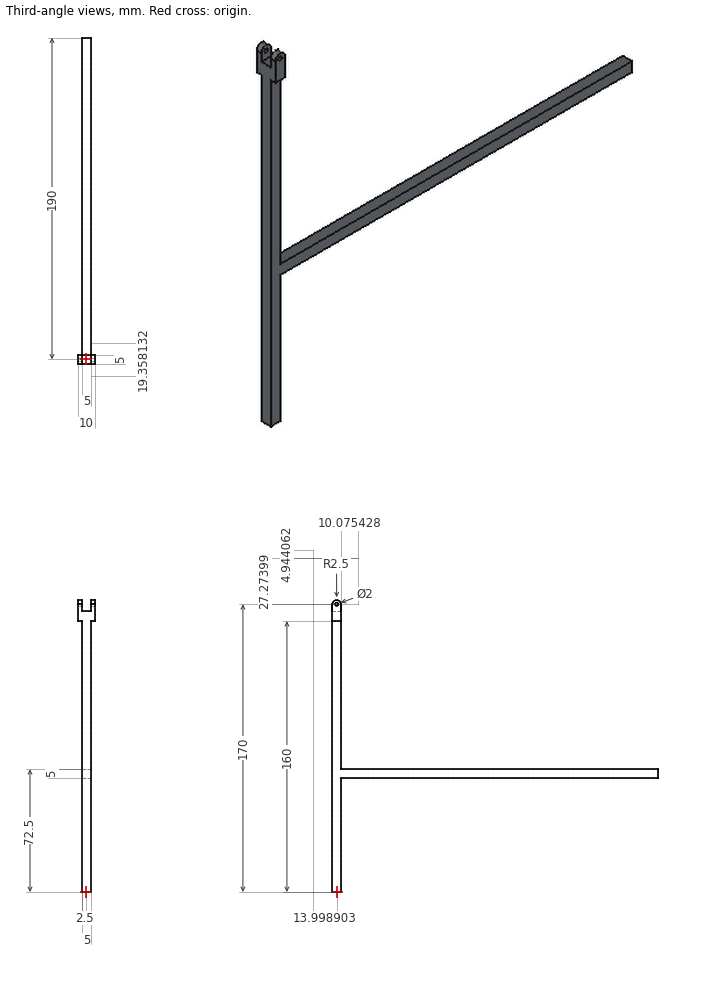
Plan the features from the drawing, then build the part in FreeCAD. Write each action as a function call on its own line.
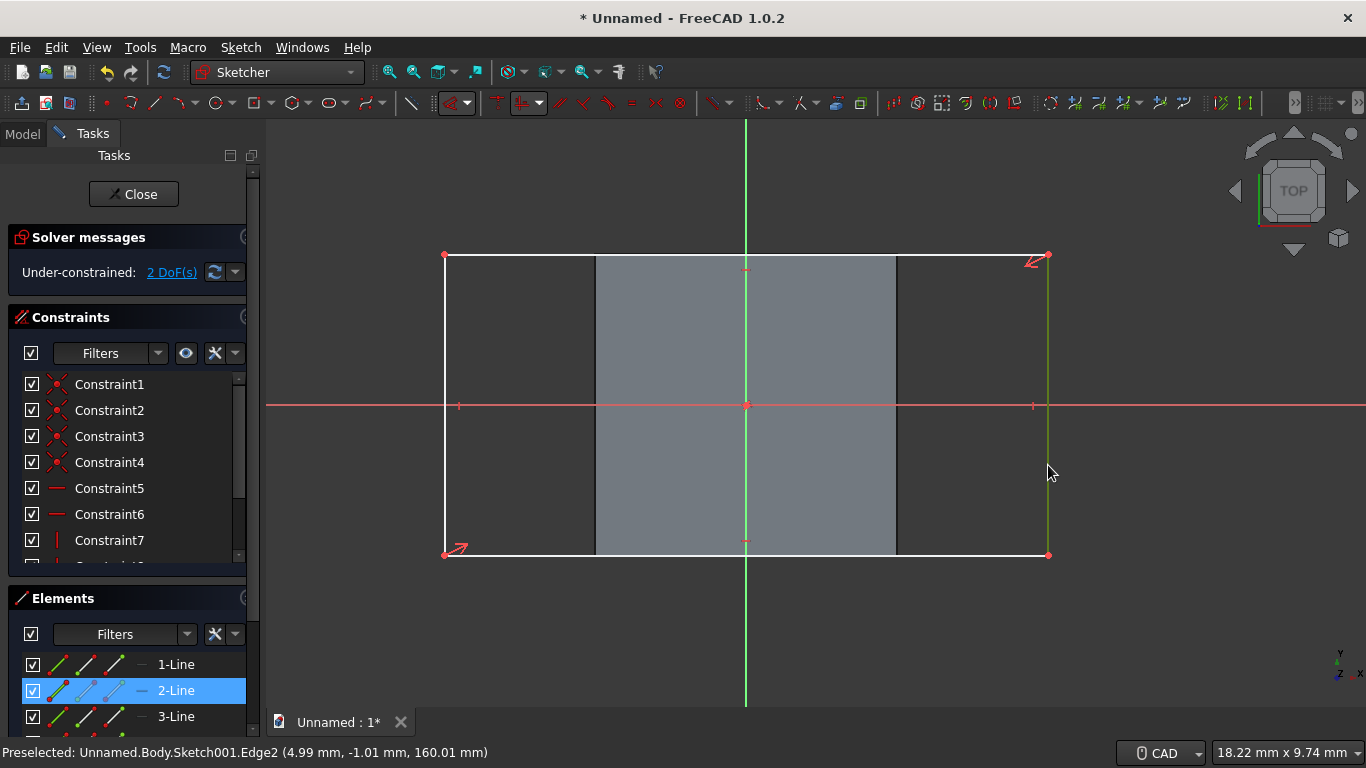
key(i)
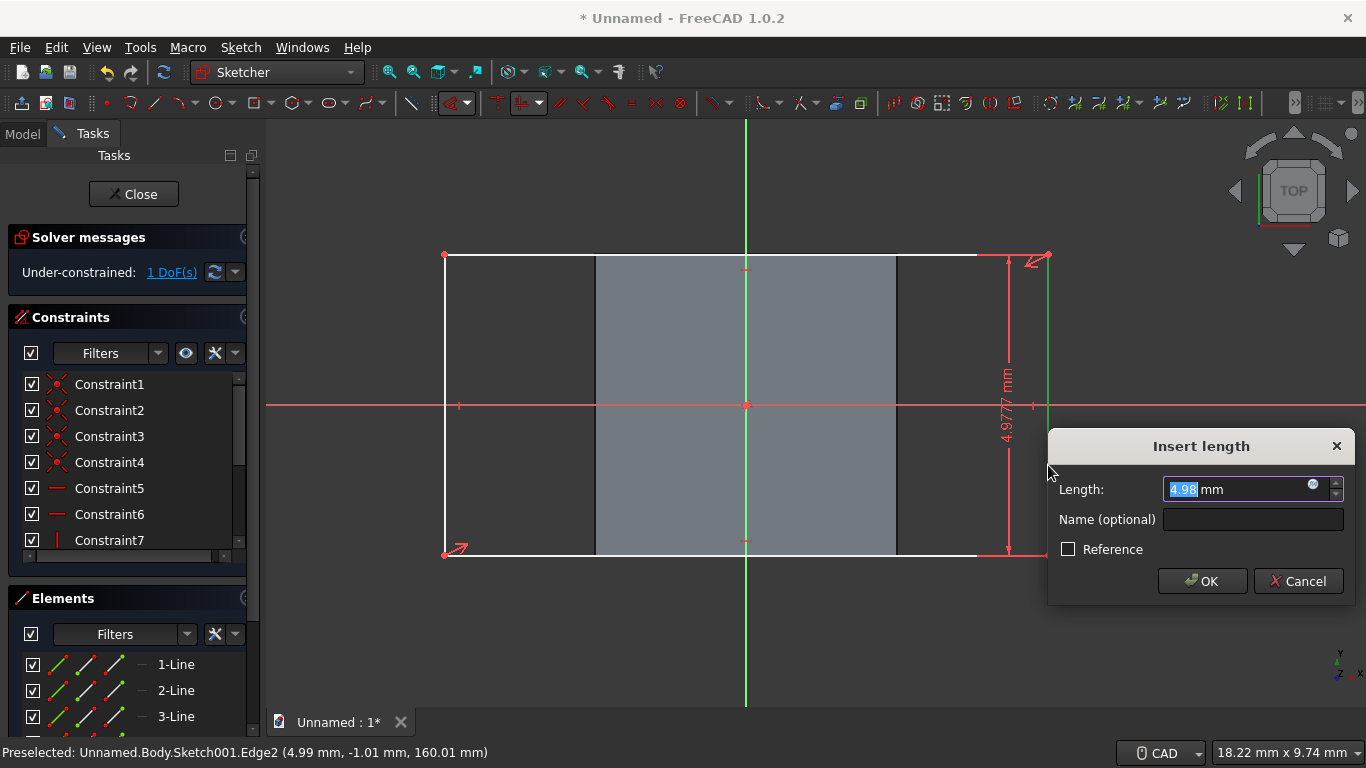
text(5)
key(Return)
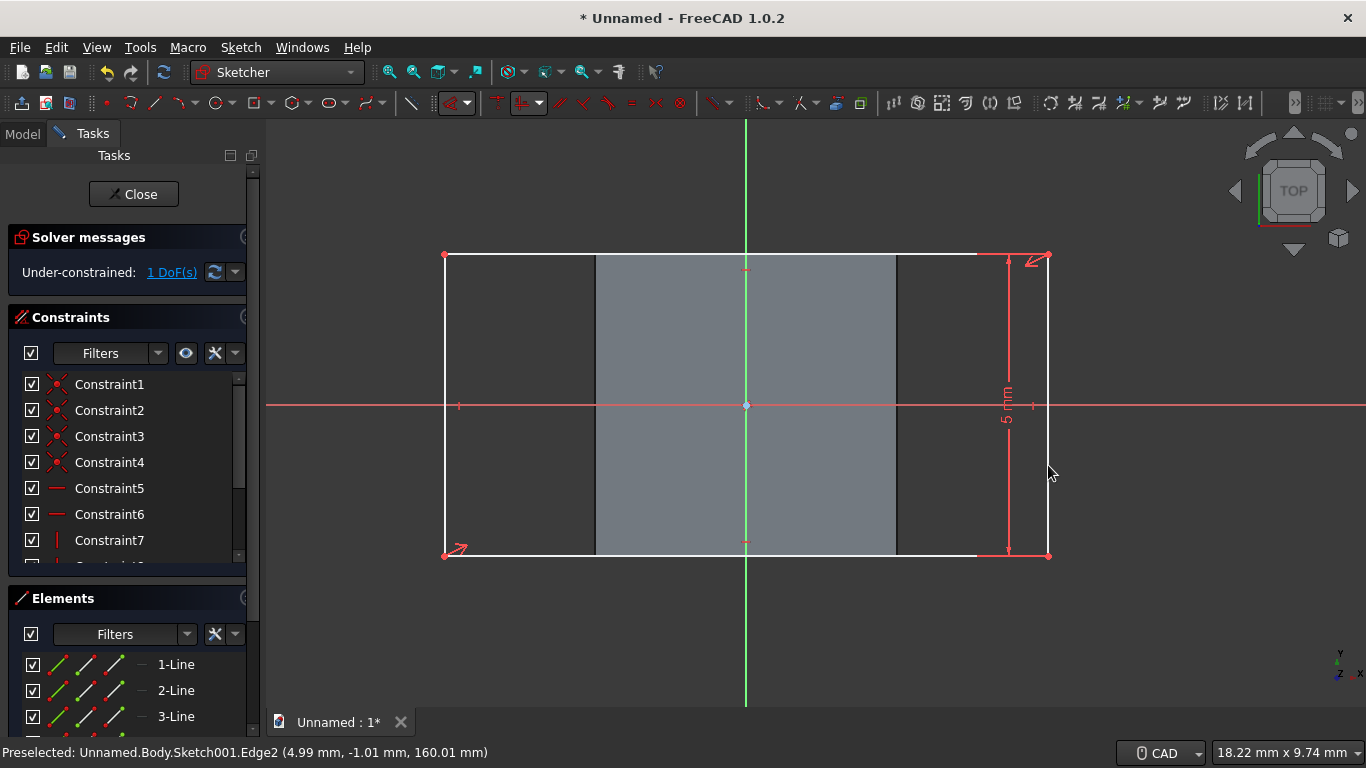
click(626, 556)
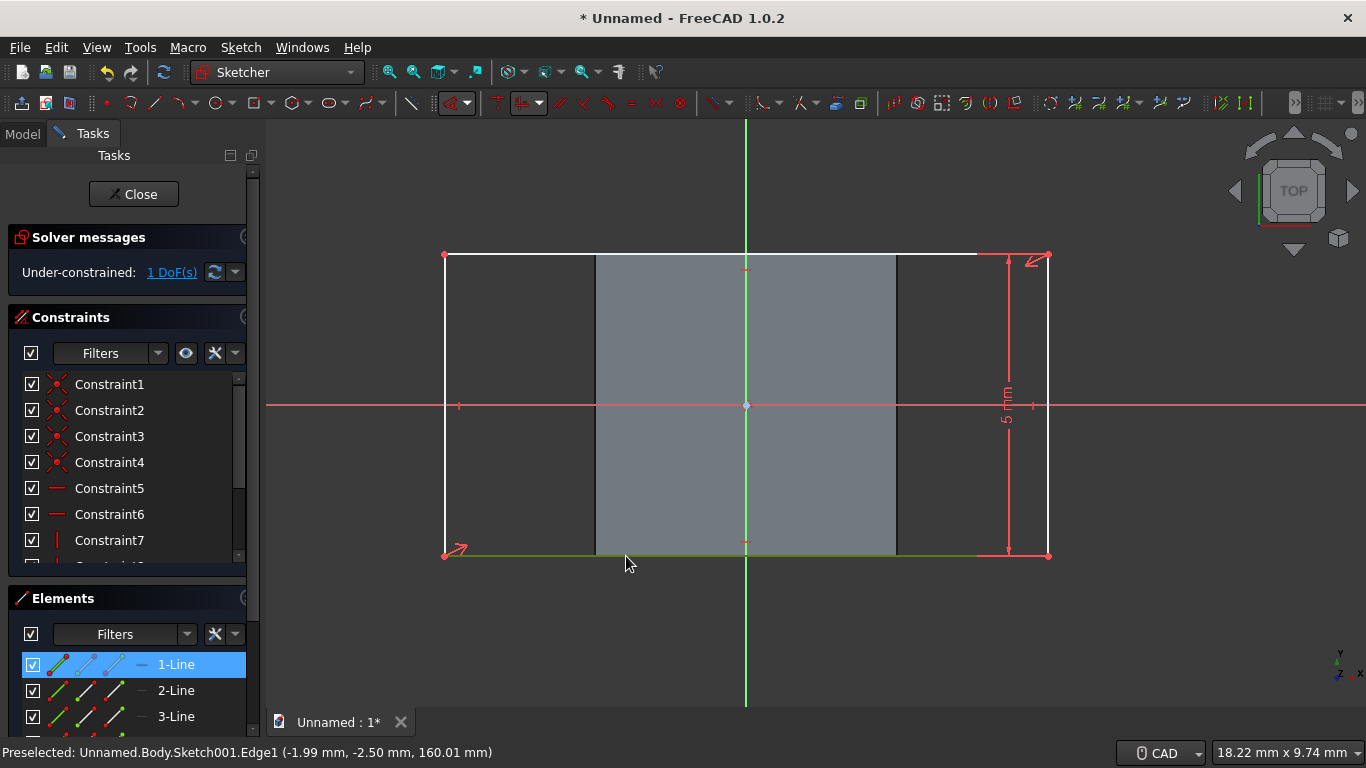
key(l)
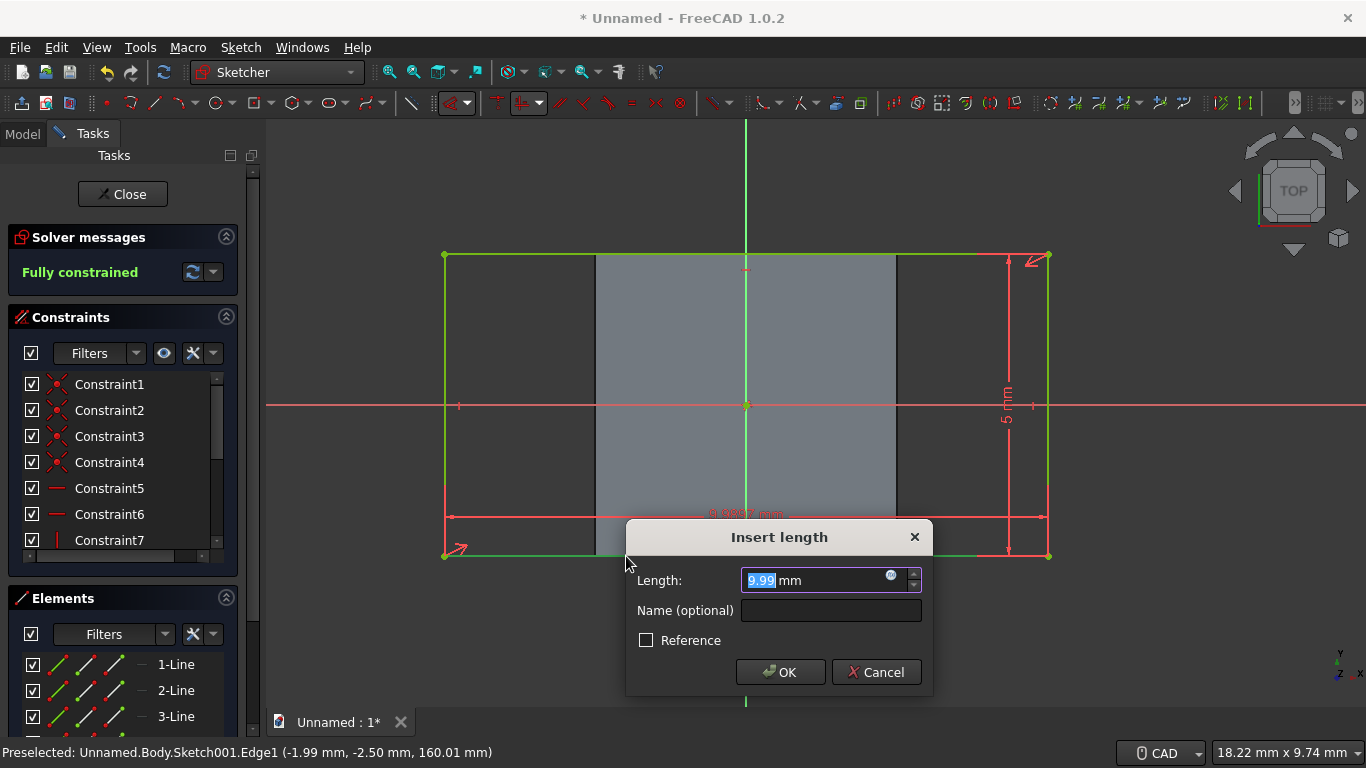
text(10)
key(Return)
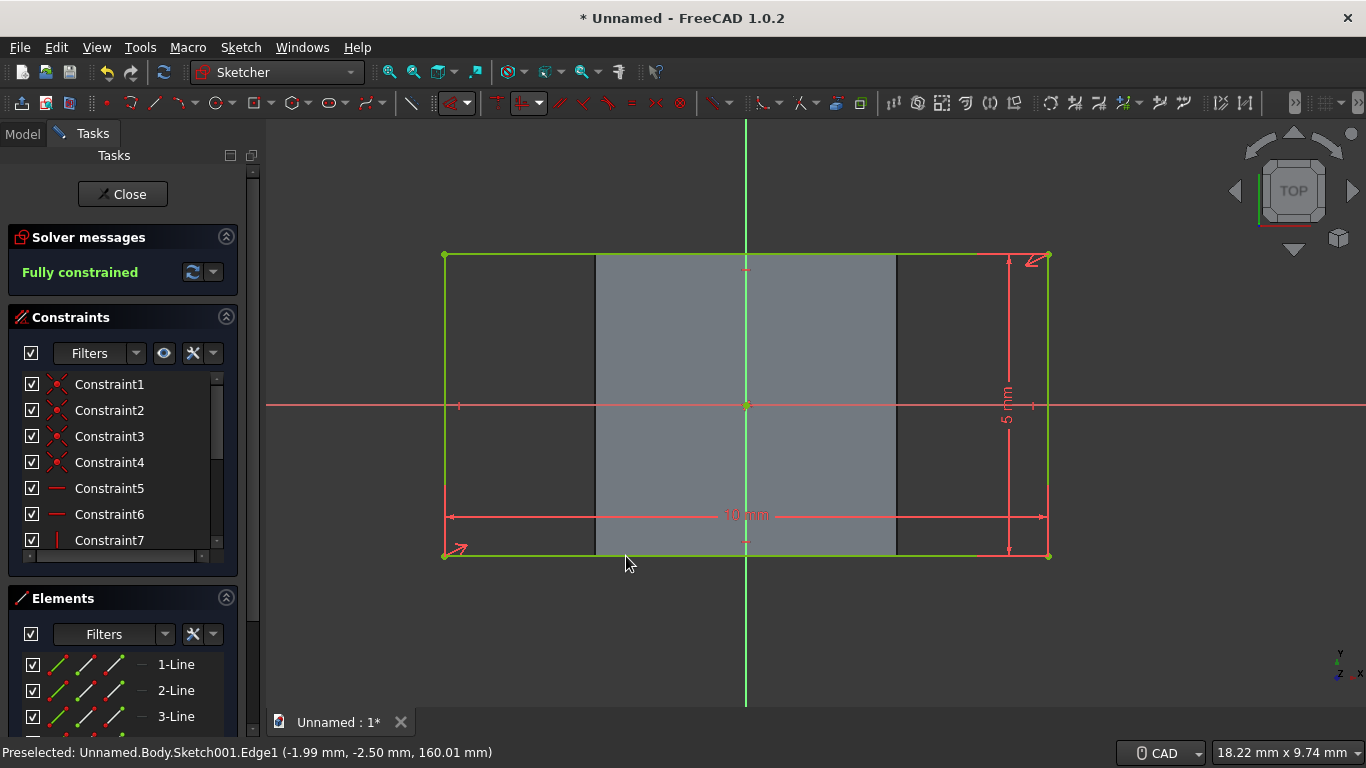
click(123, 194)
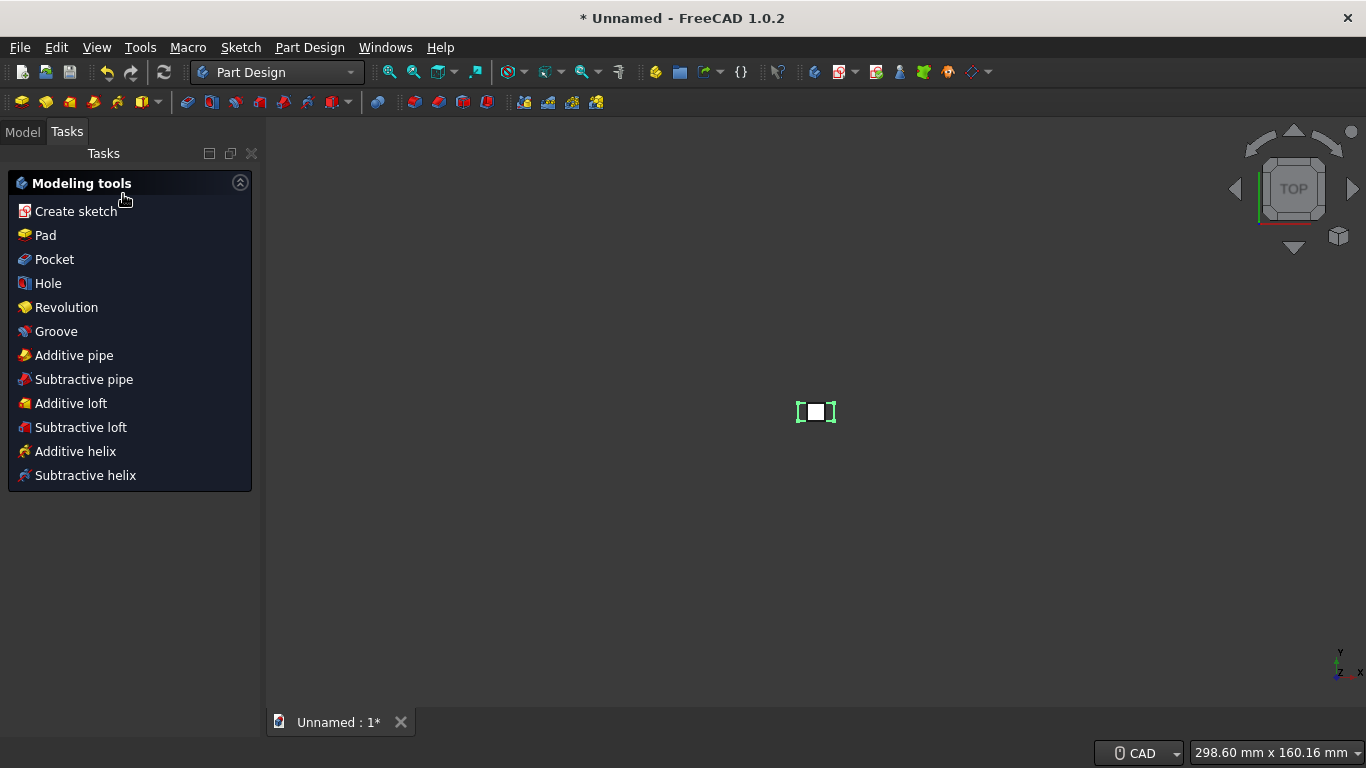
click(22, 102)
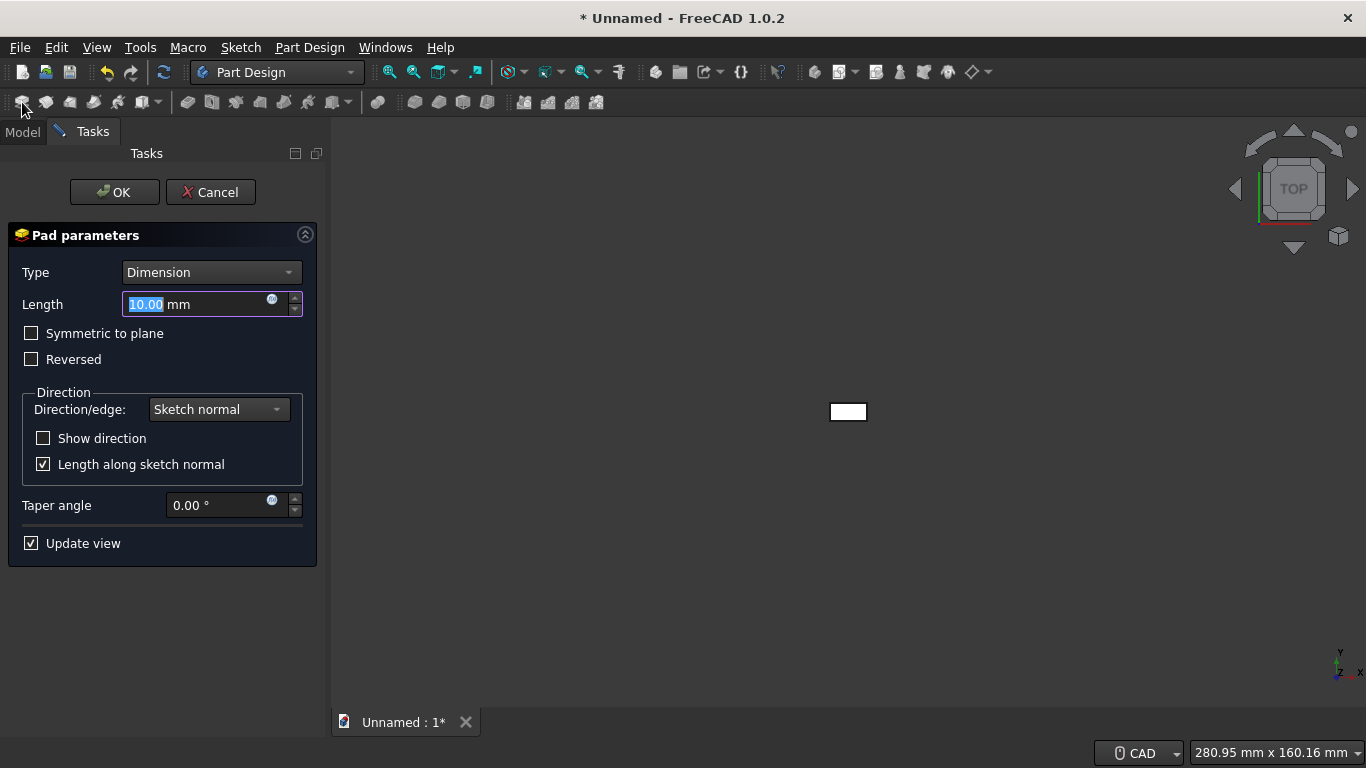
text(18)
key(Tab)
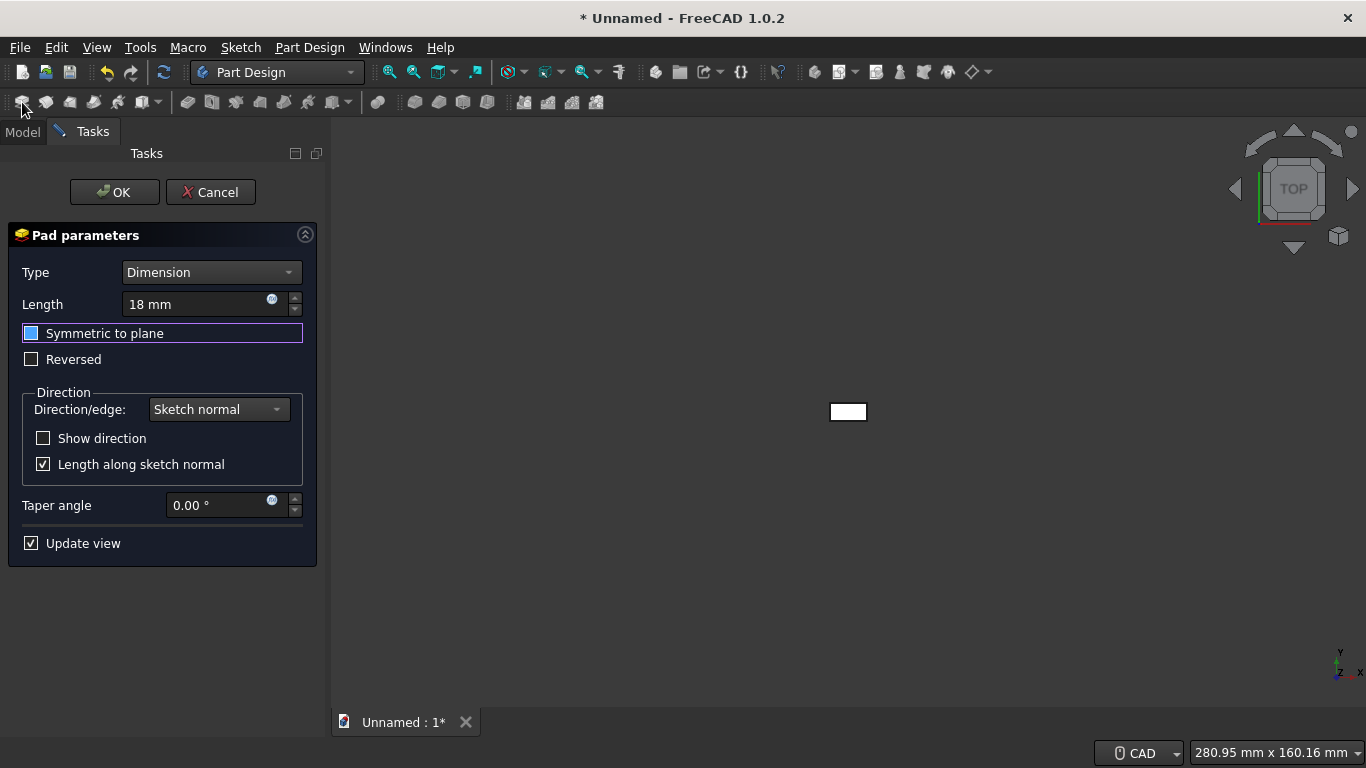
click(115, 192)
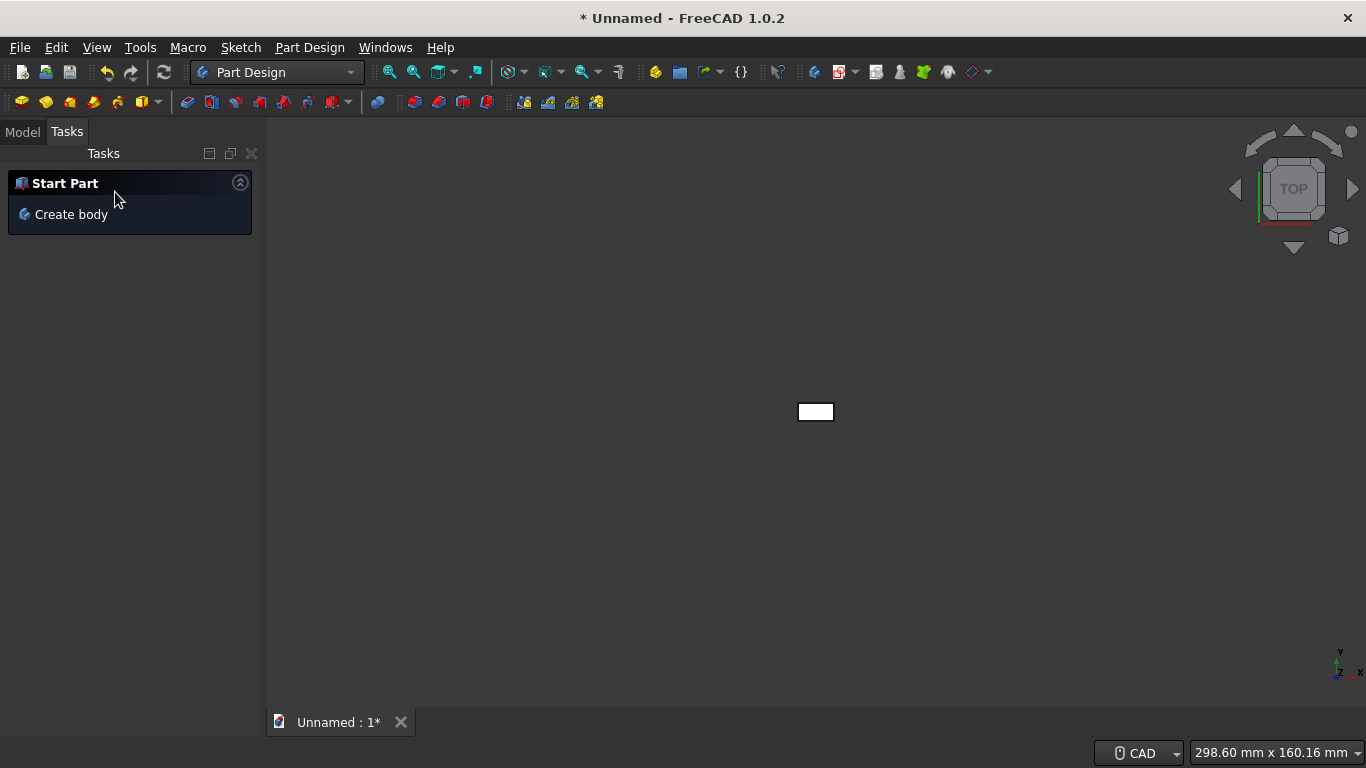
click(390, 72)